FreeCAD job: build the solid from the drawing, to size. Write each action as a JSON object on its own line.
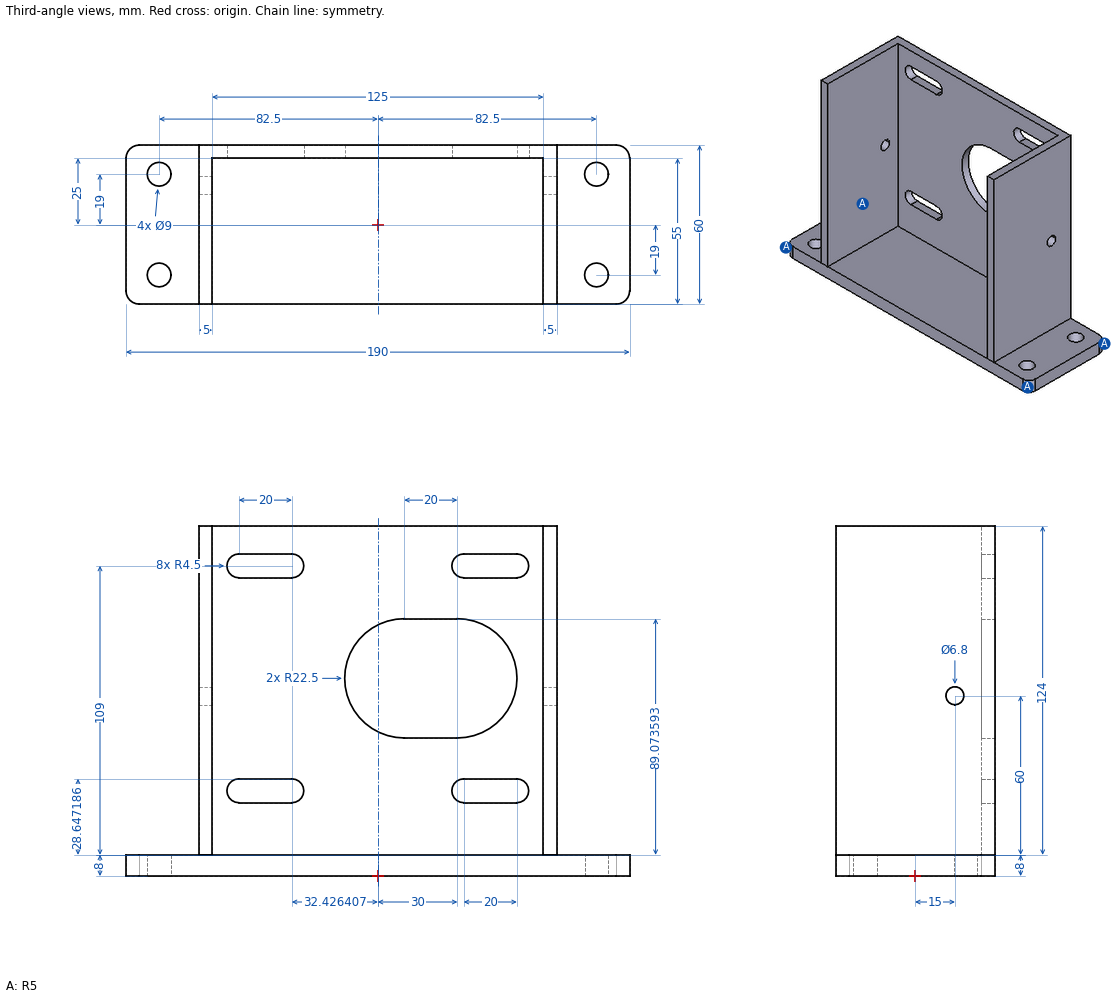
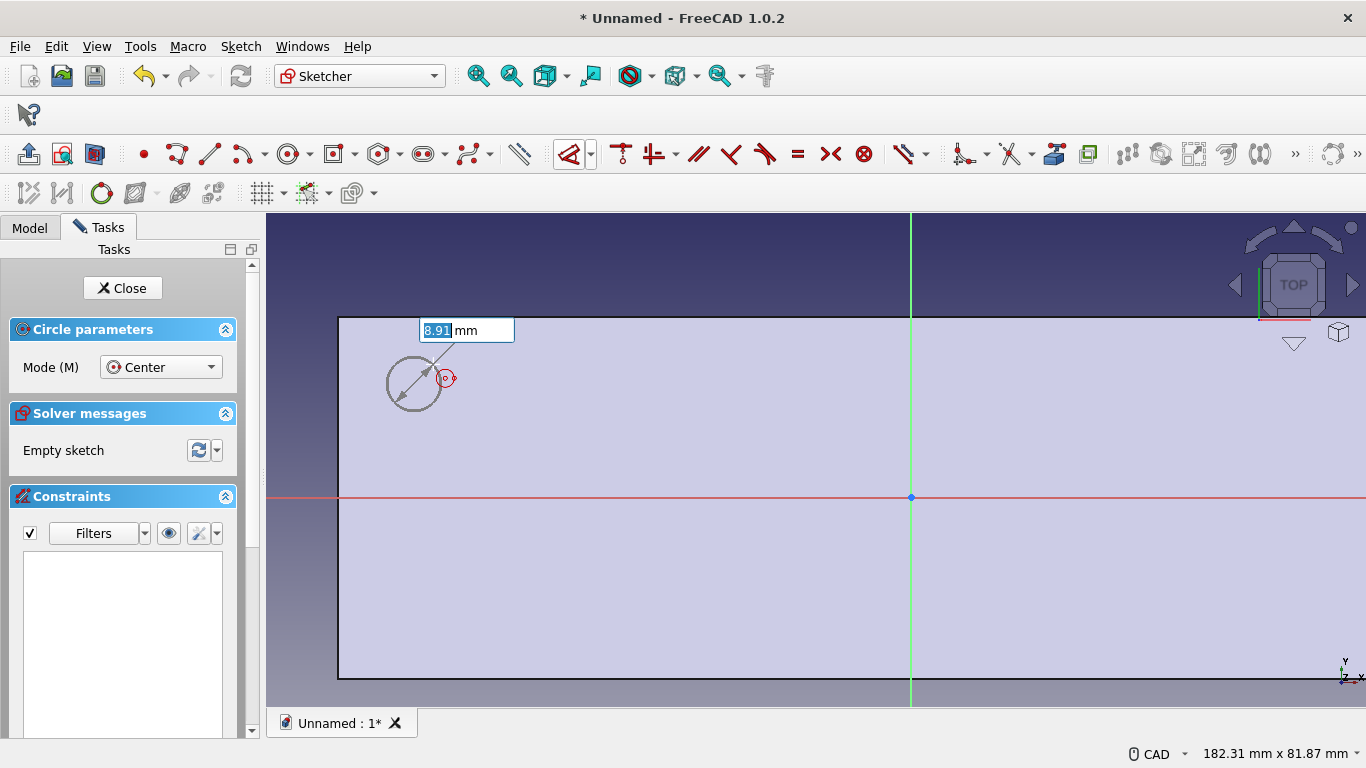
{"action": "type", "text": "9"}
{"action": "key", "text": "Return"}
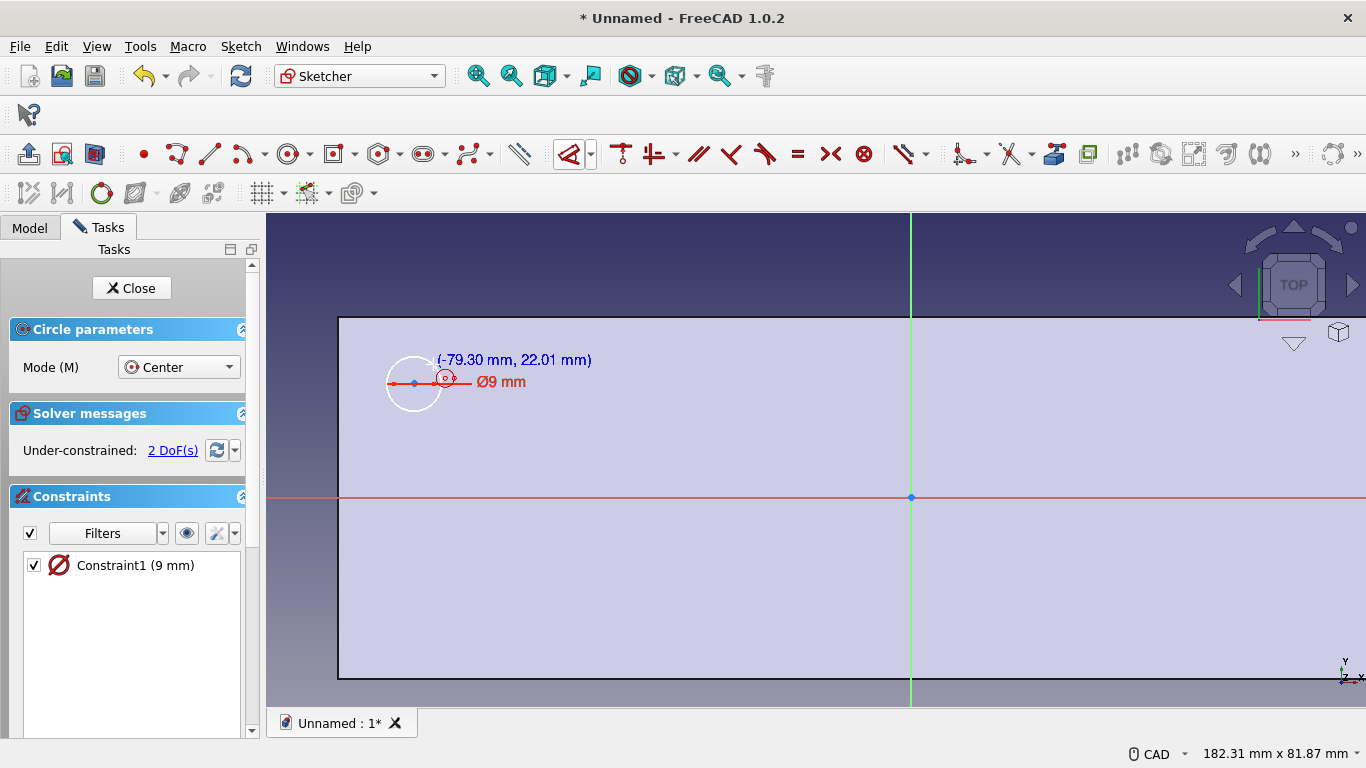
{"action": "scroll", "coordinate": [414, 383], "scroll_direction": "down", "scroll_amount": 2}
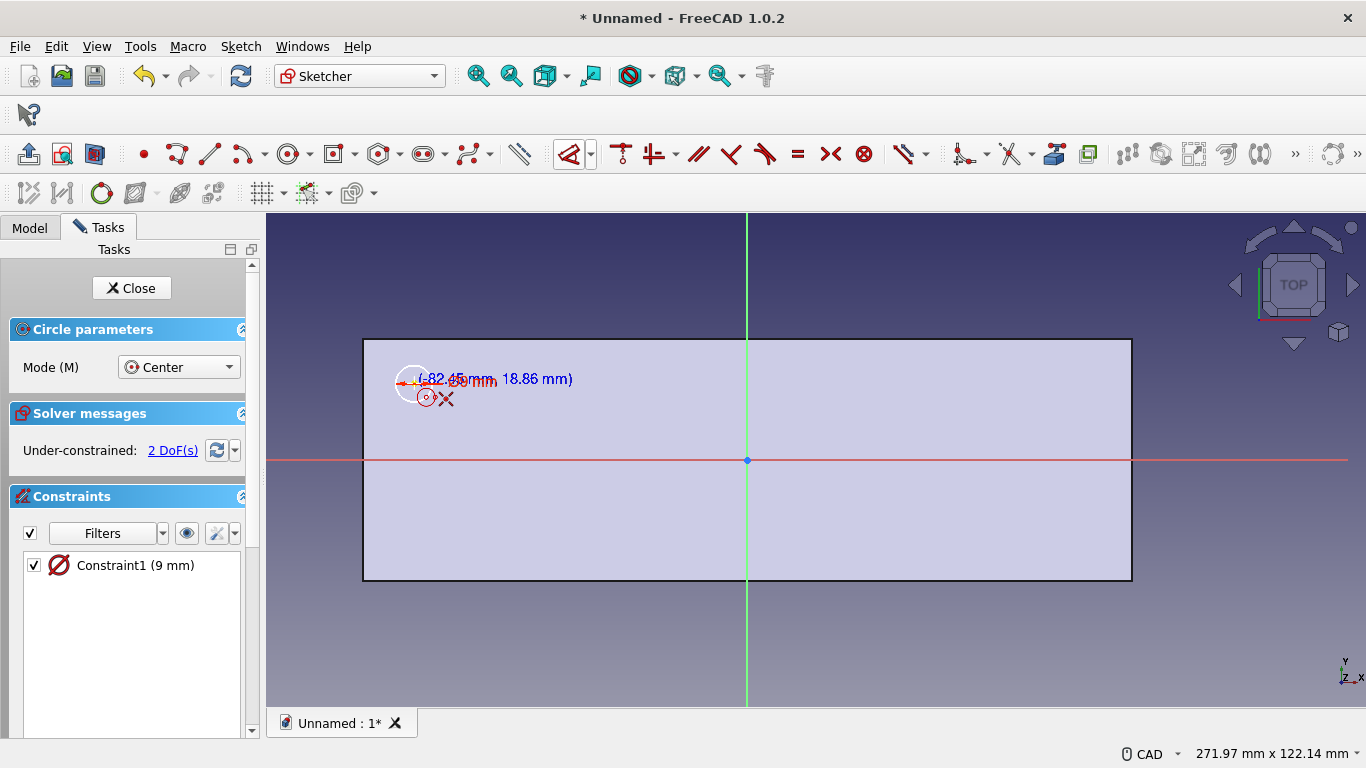
{"action": "scroll", "coordinate": [1081, 383], "scroll_direction": "up", "scroll_amount": 2}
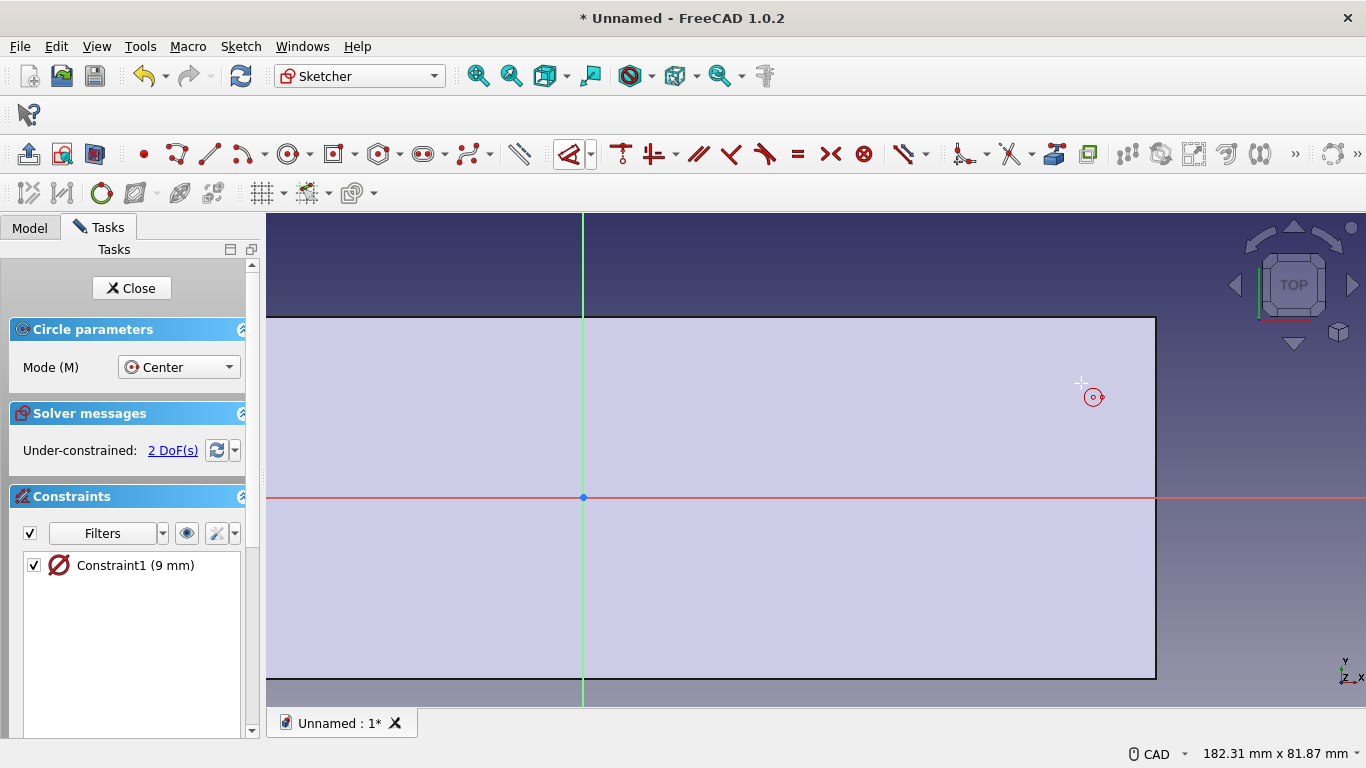
{"action": "left_click", "coordinate": [1081, 383]}
{"action": "mouse_move", "coordinate": [1100, 364]}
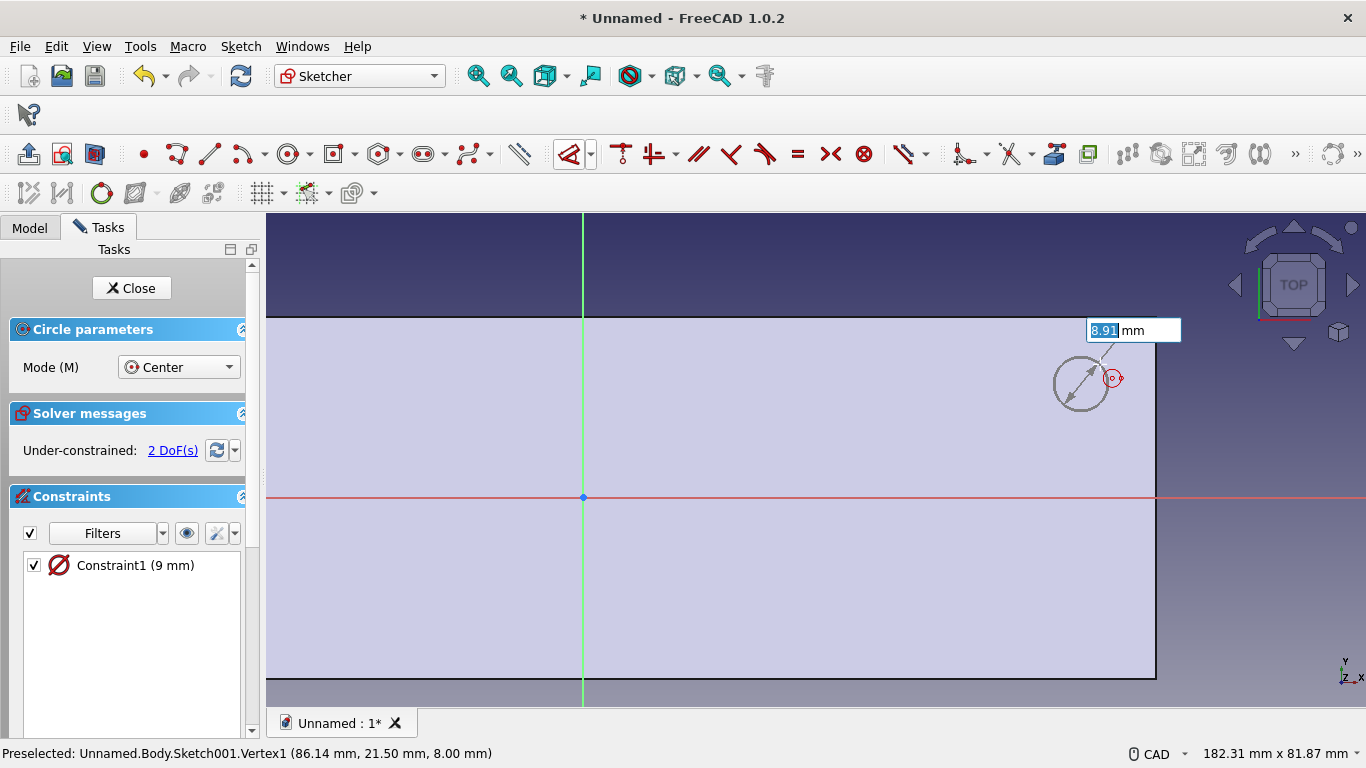
{"action": "type", "text": "9"}
{"action": "key", "text": "Return"}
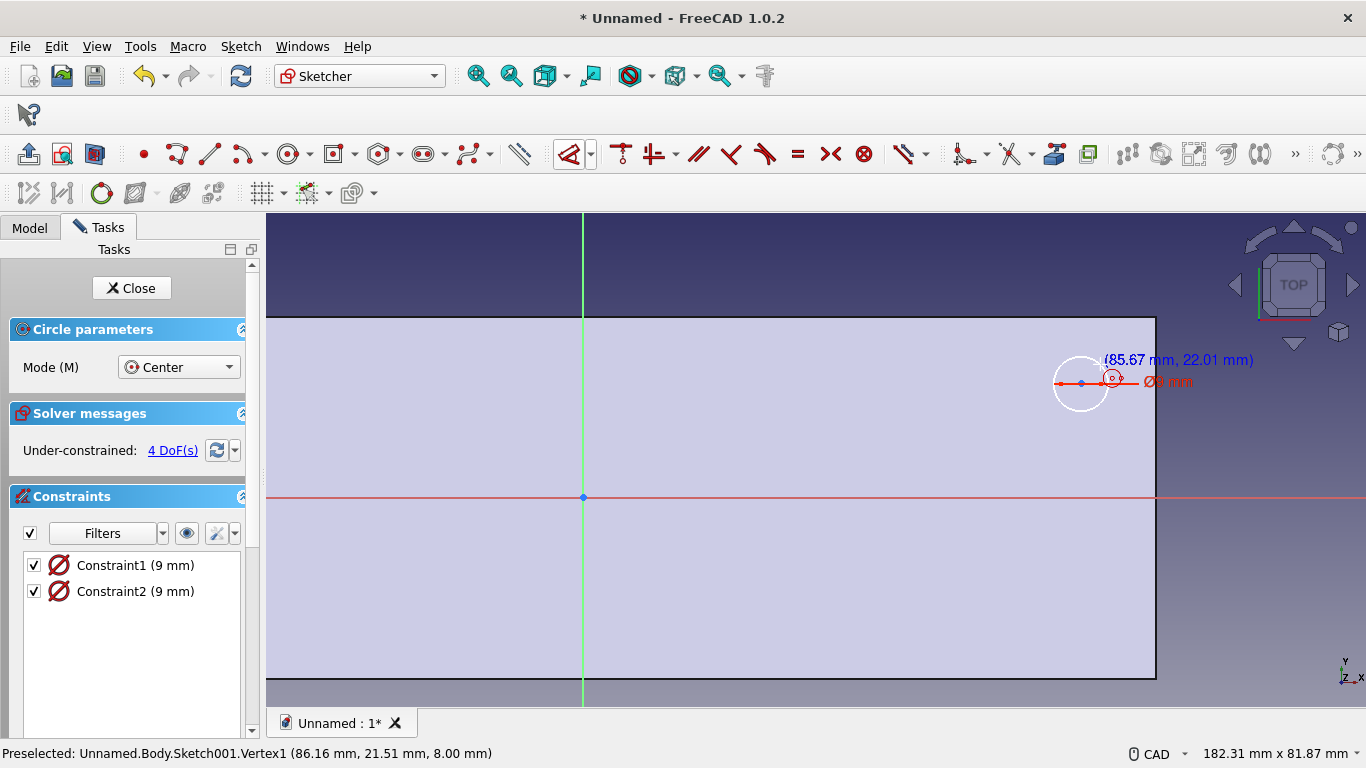
{"action": "left_click", "coordinate": [1081, 612]}
{"action": "mouse_move", "coordinate": [1100, 593]}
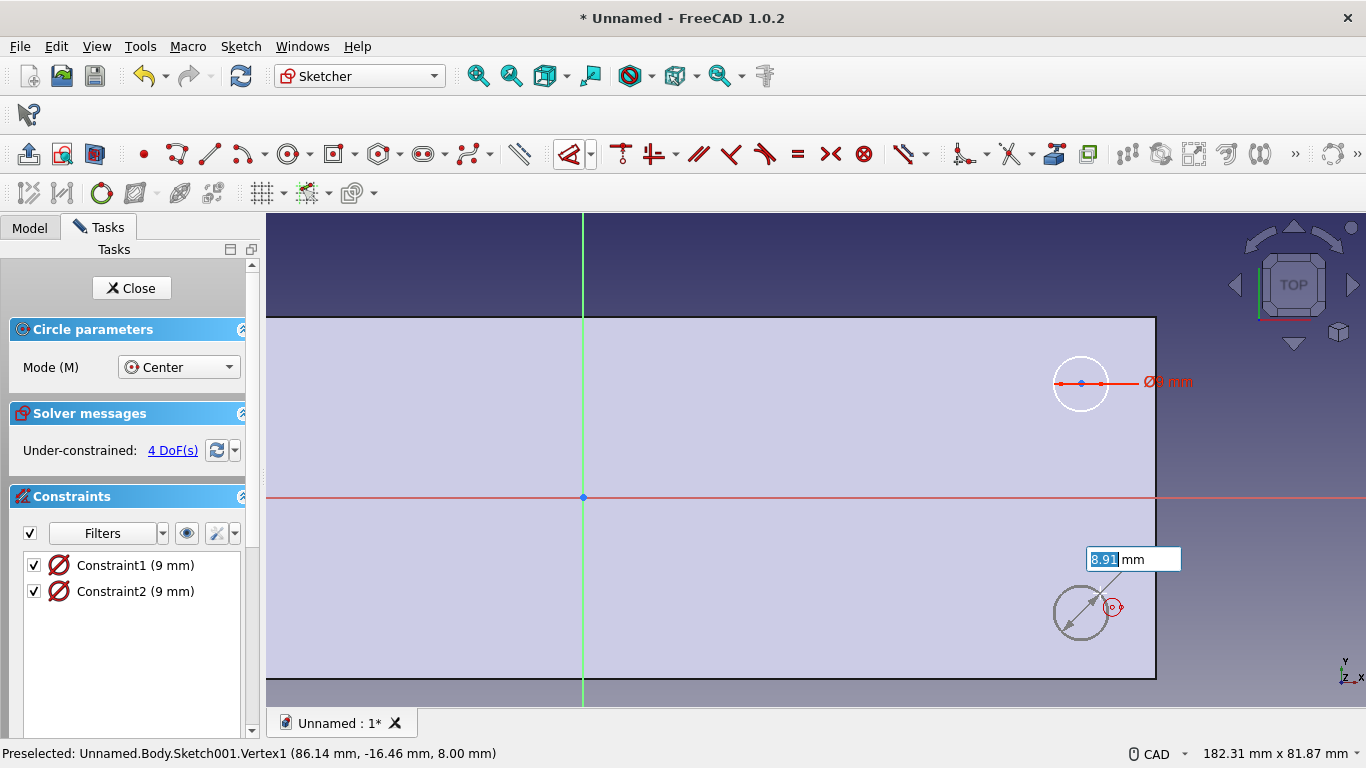
{"action": "type", "text": "9"}
{"action": "key", "text": "Return"}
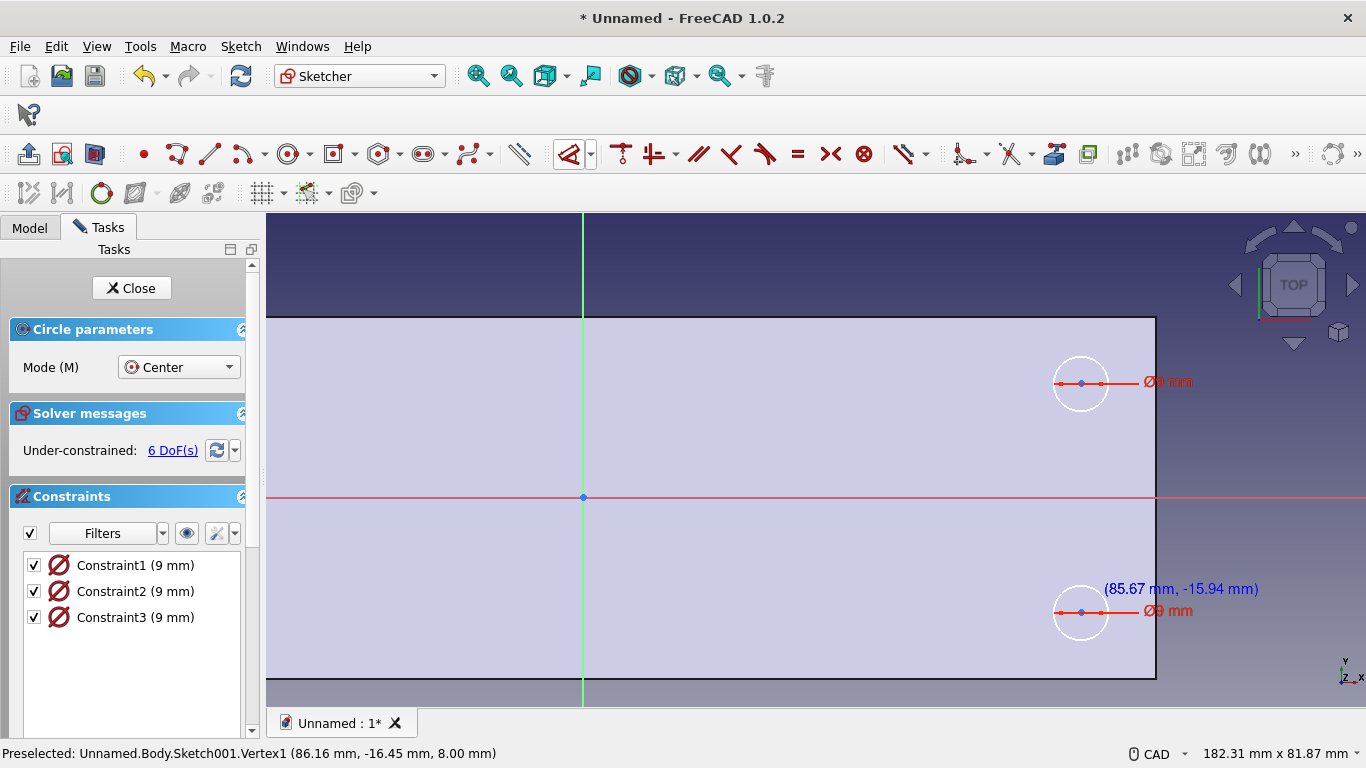
{"action": "scroll", "coordinate": [1082, 383], "scroll_direction": "down", "scroll_amount": 2}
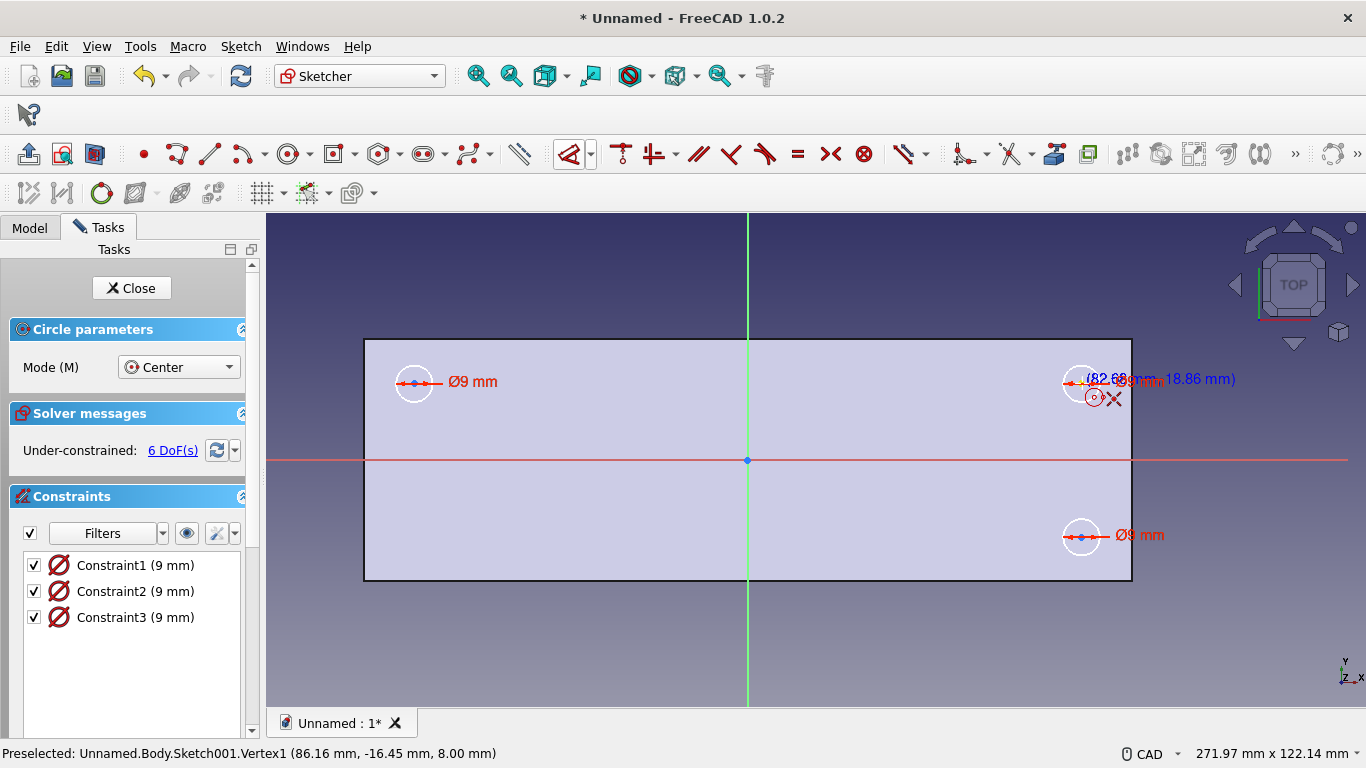
{"action": "scroll", "coordinate": [414, 537], "scroll_direction": "up", "scroll_amount": 2}